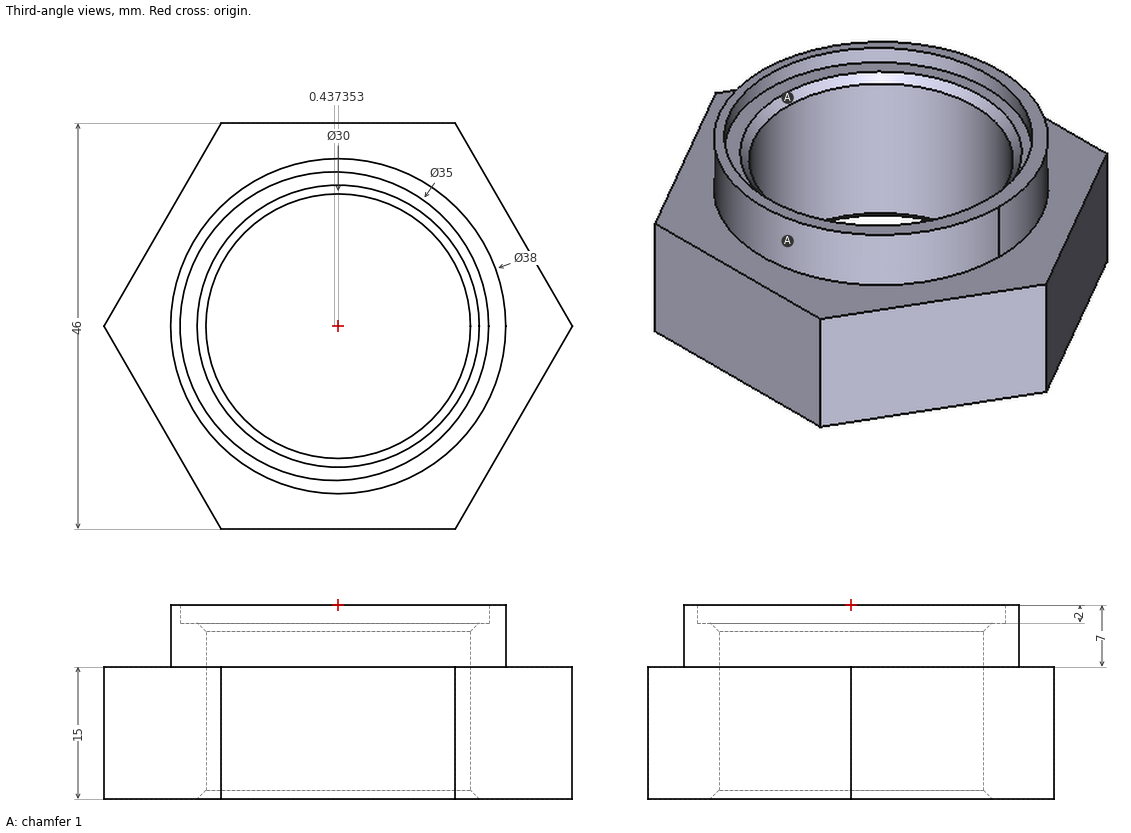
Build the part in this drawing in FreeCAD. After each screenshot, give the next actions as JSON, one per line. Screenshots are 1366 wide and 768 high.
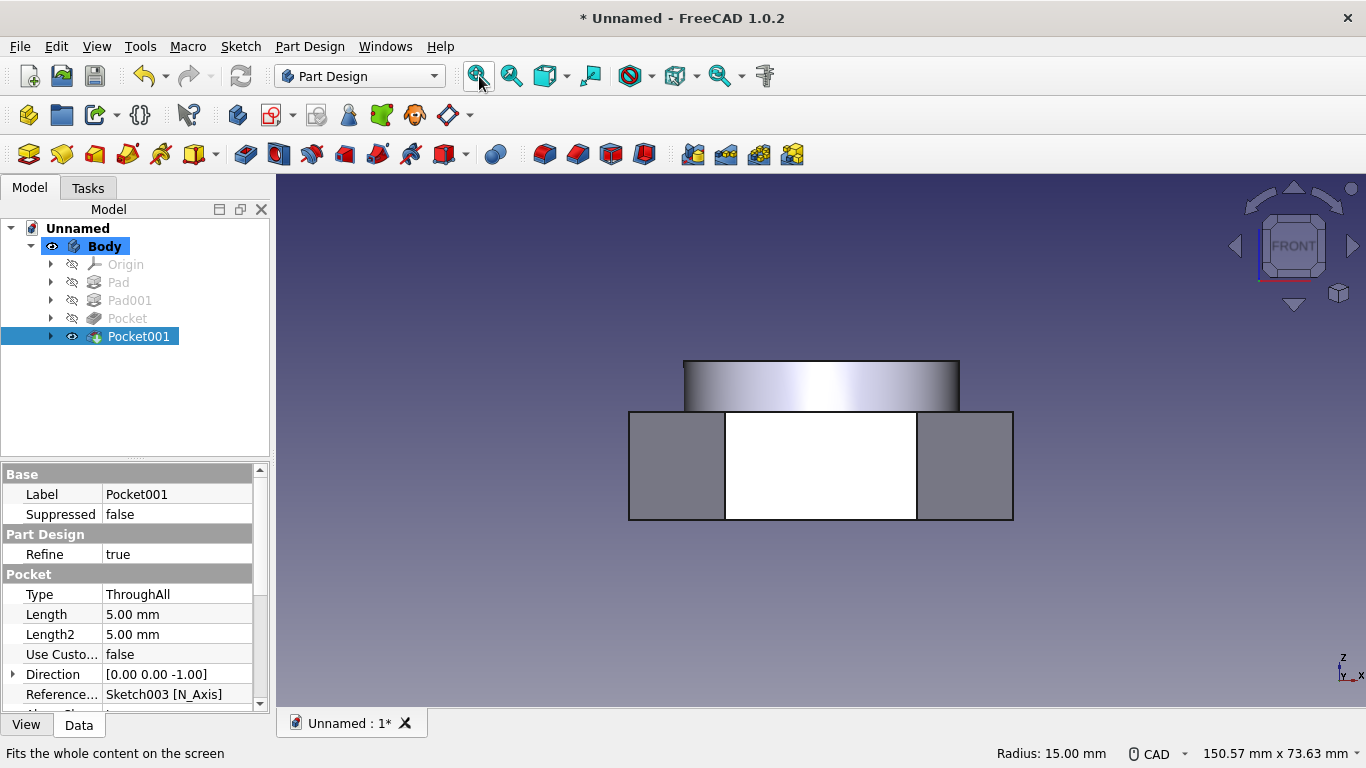
{"action": "key", "text": "3"}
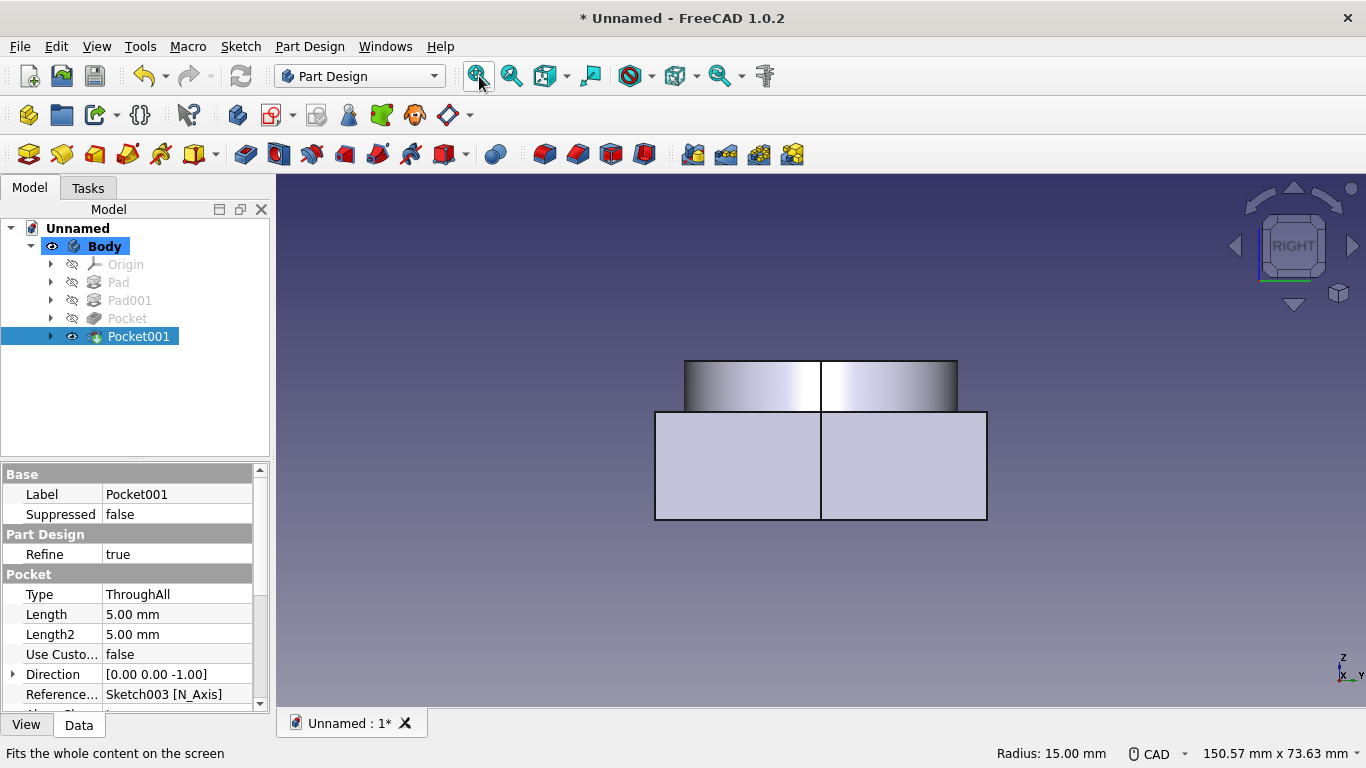
{"action": "left_click", "coordinate": [479, 76]}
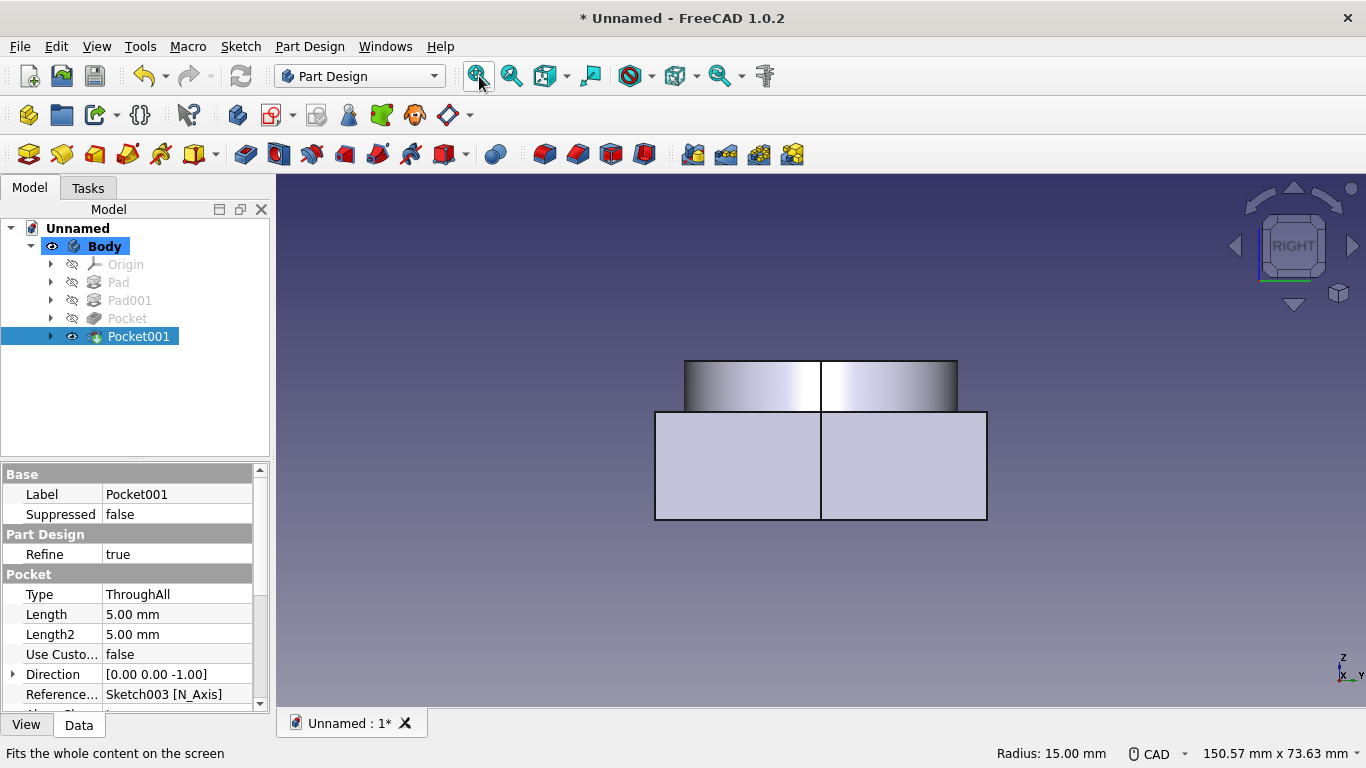
{"action": "key", "text": "5"}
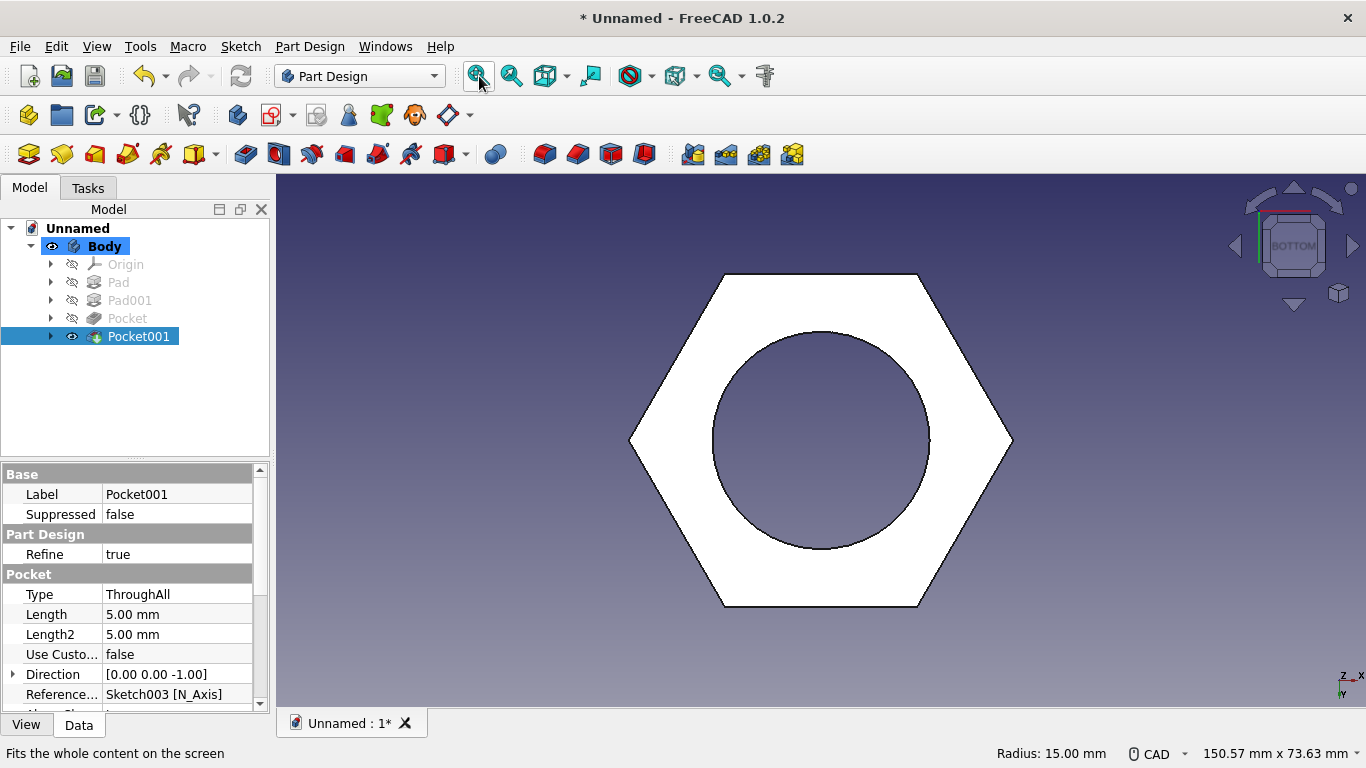
{"action": "left_click", "coordinate": [712, 439], "text": "ctrl"}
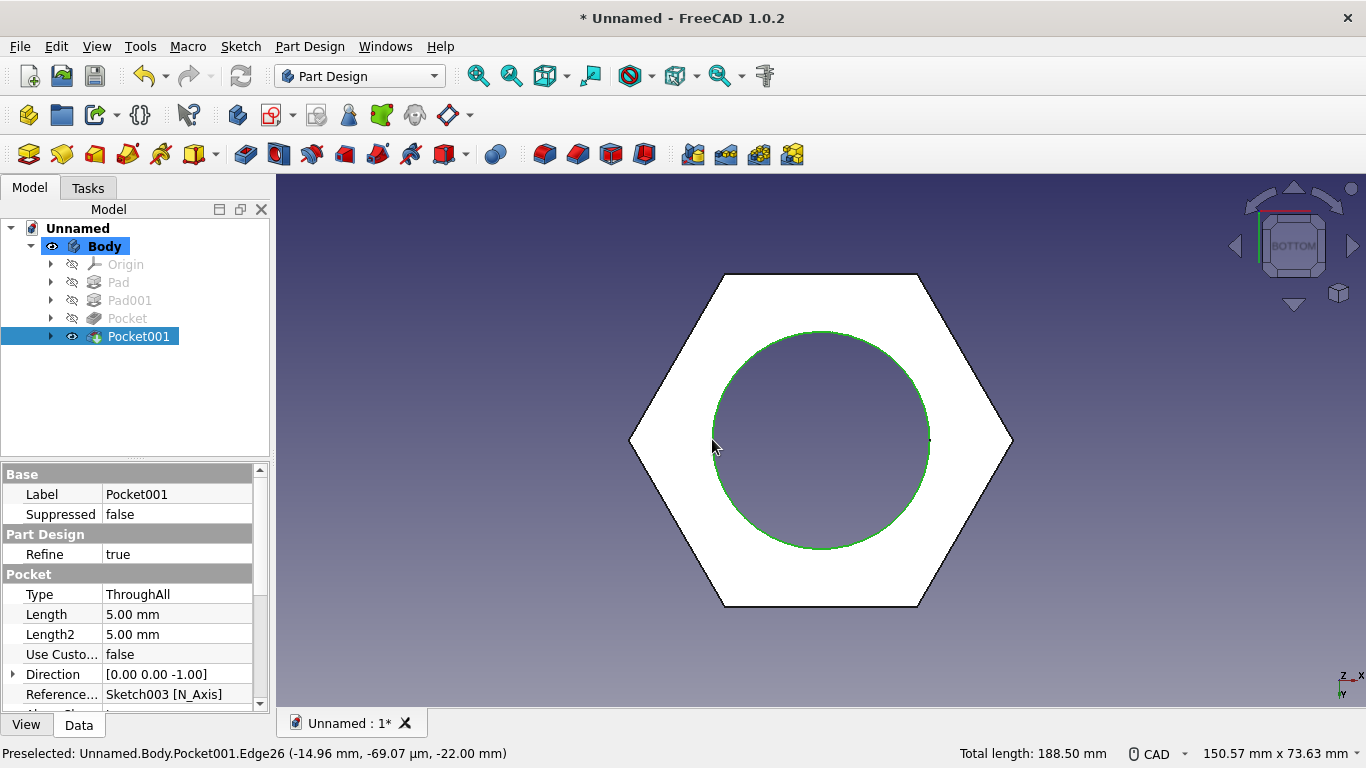
{"action": "left_click", "coordinate": [578, 154]}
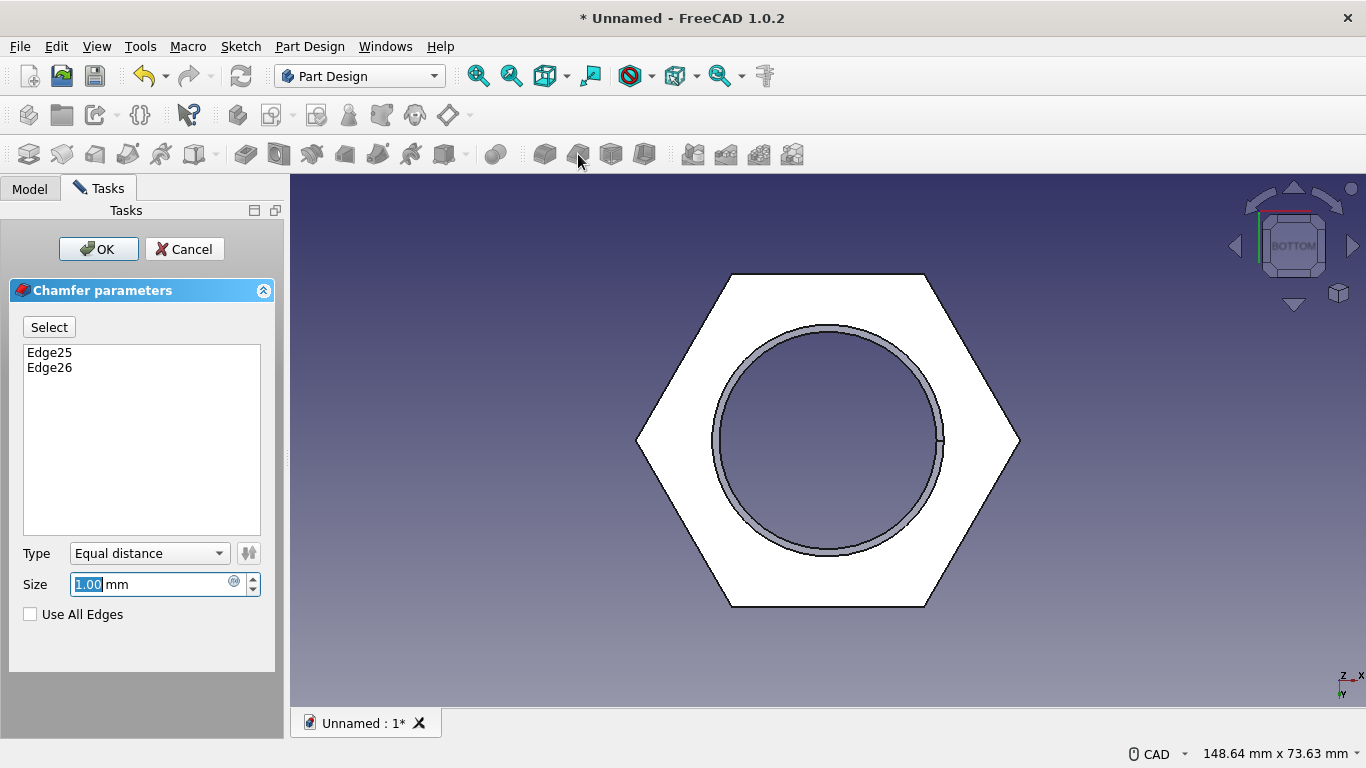
{"action": "type", "text": "1"}
{"action": "key", "text": "Tab"}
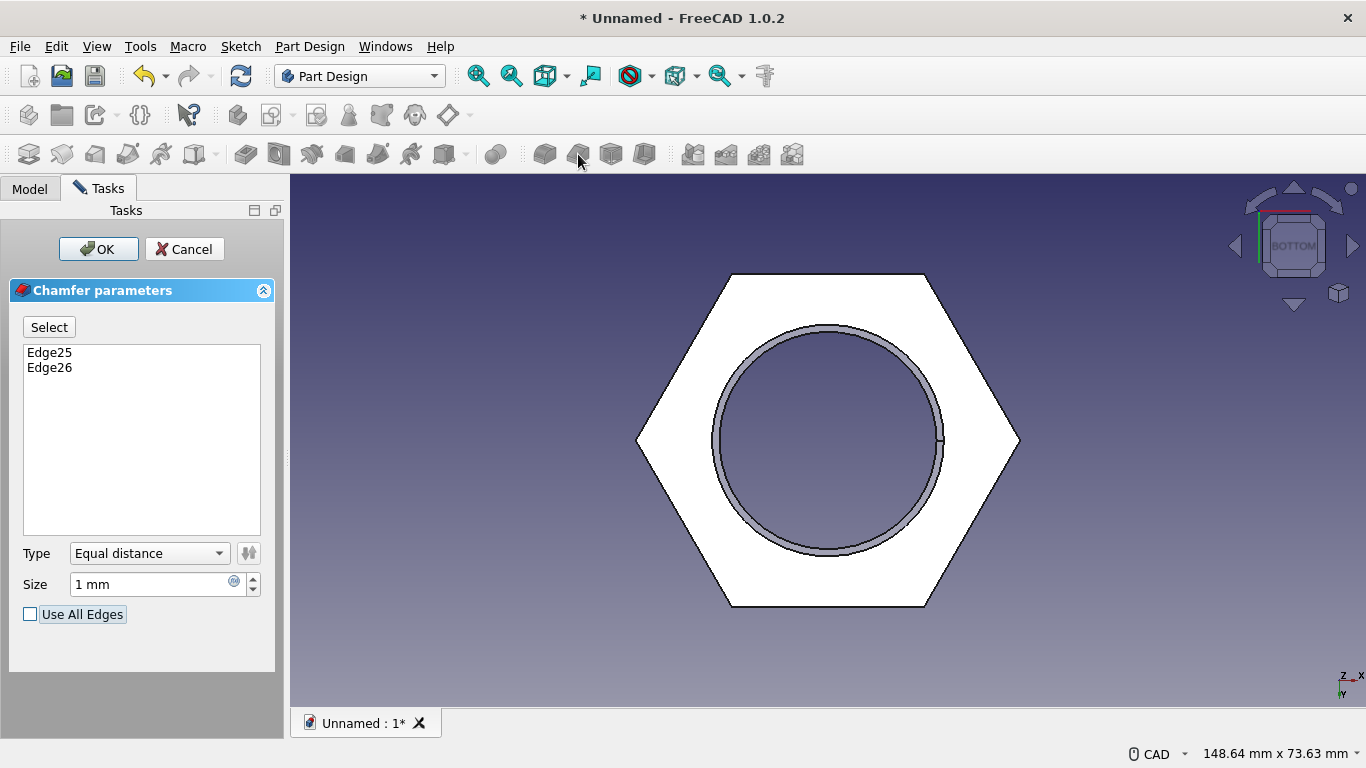
{"action": "left_click", "coordinate": [99, 249]}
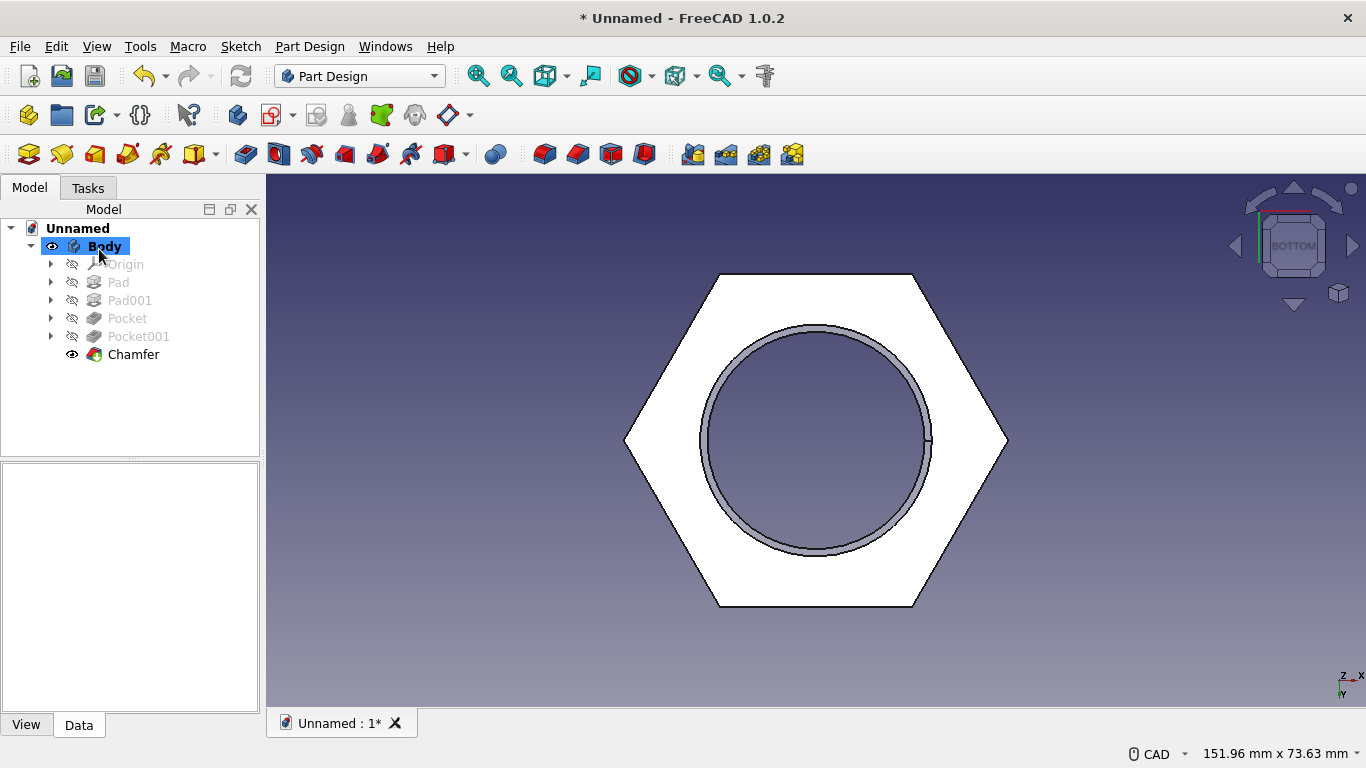
{"action": "key", "text": "0"}